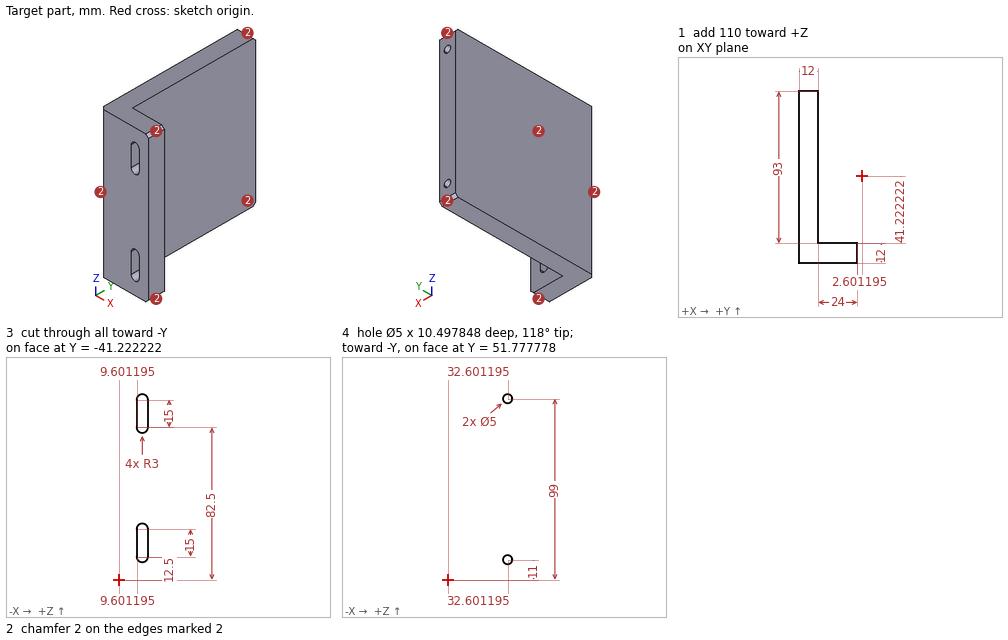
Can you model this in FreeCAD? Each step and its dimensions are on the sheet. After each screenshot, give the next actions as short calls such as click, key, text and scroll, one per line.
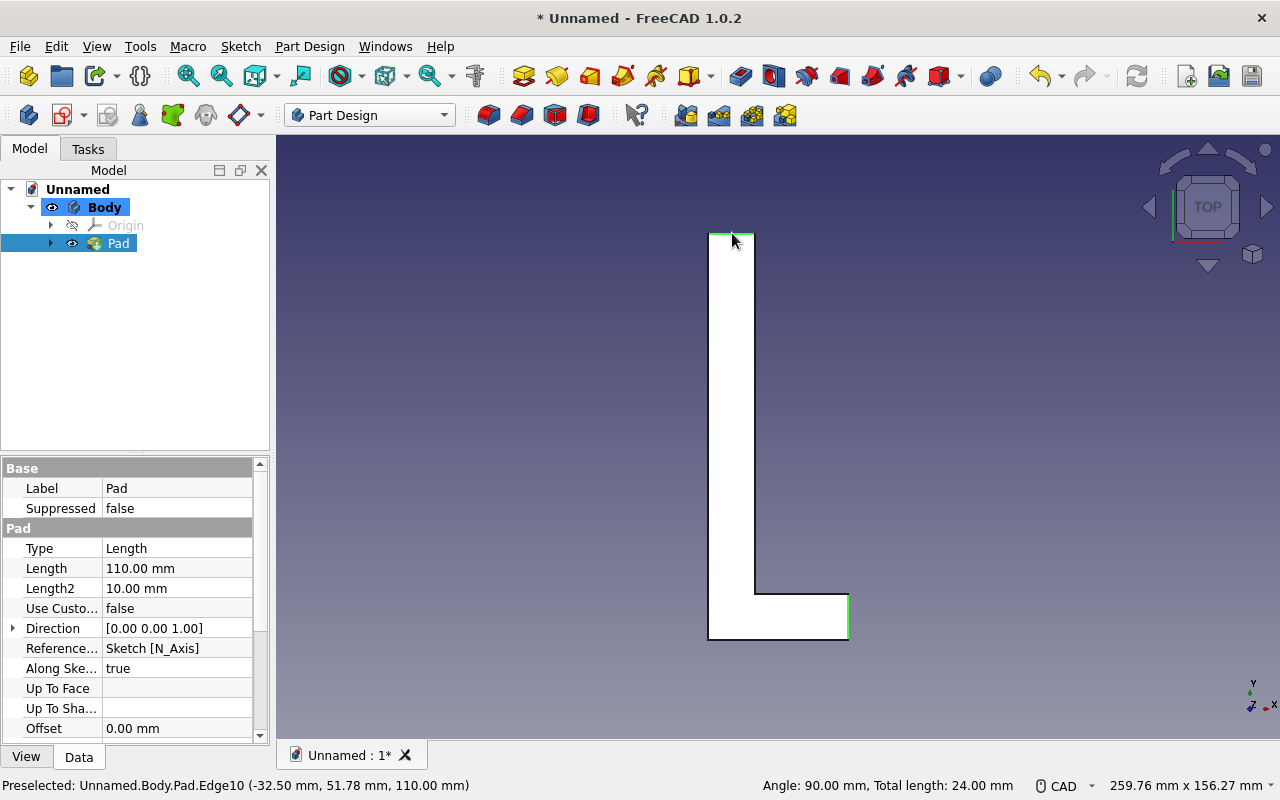
key(1)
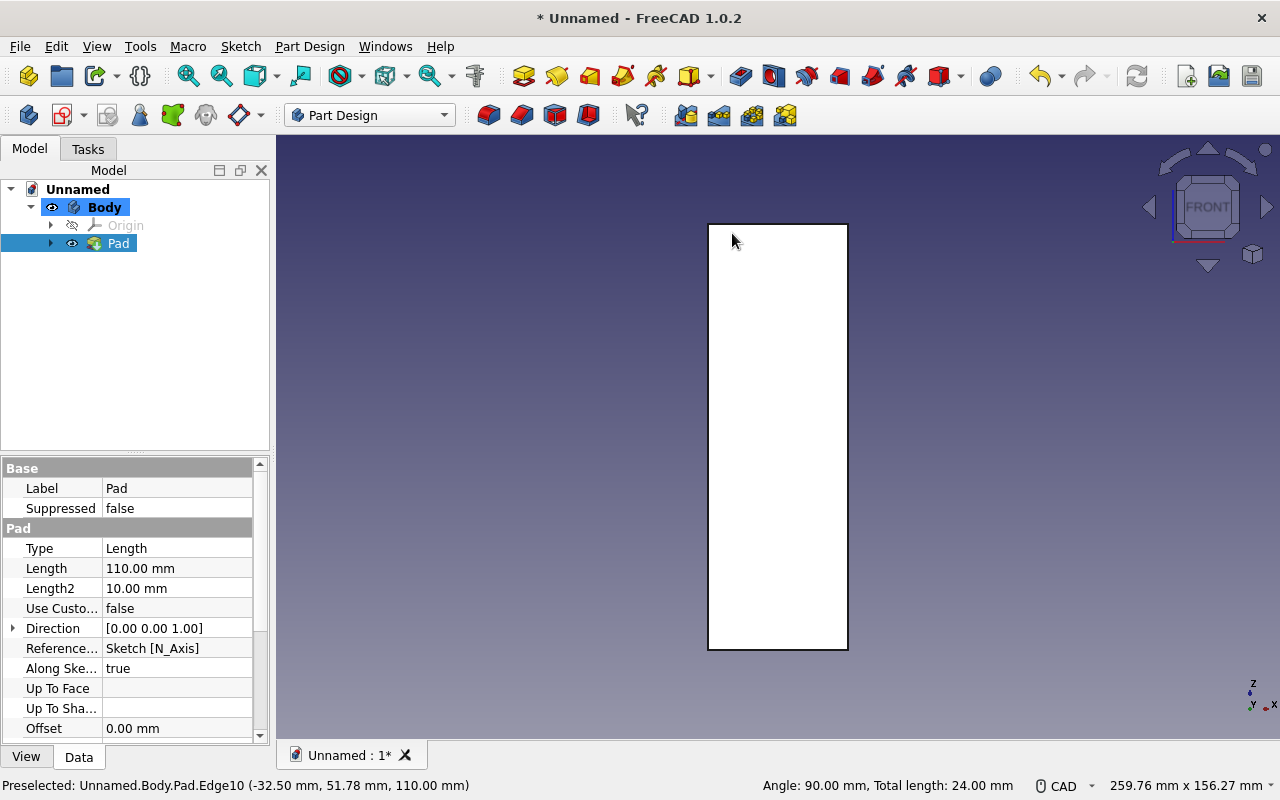
click(708, 436, ctrl)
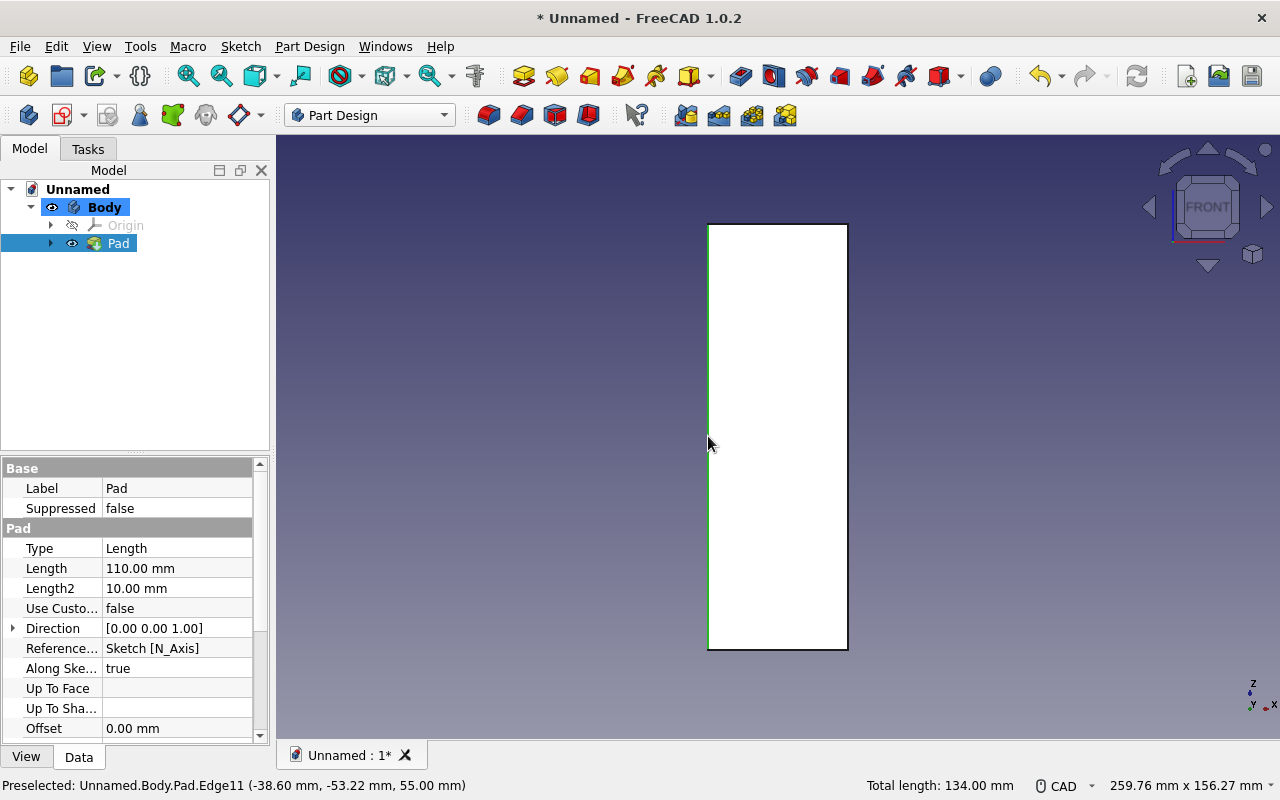
key(3)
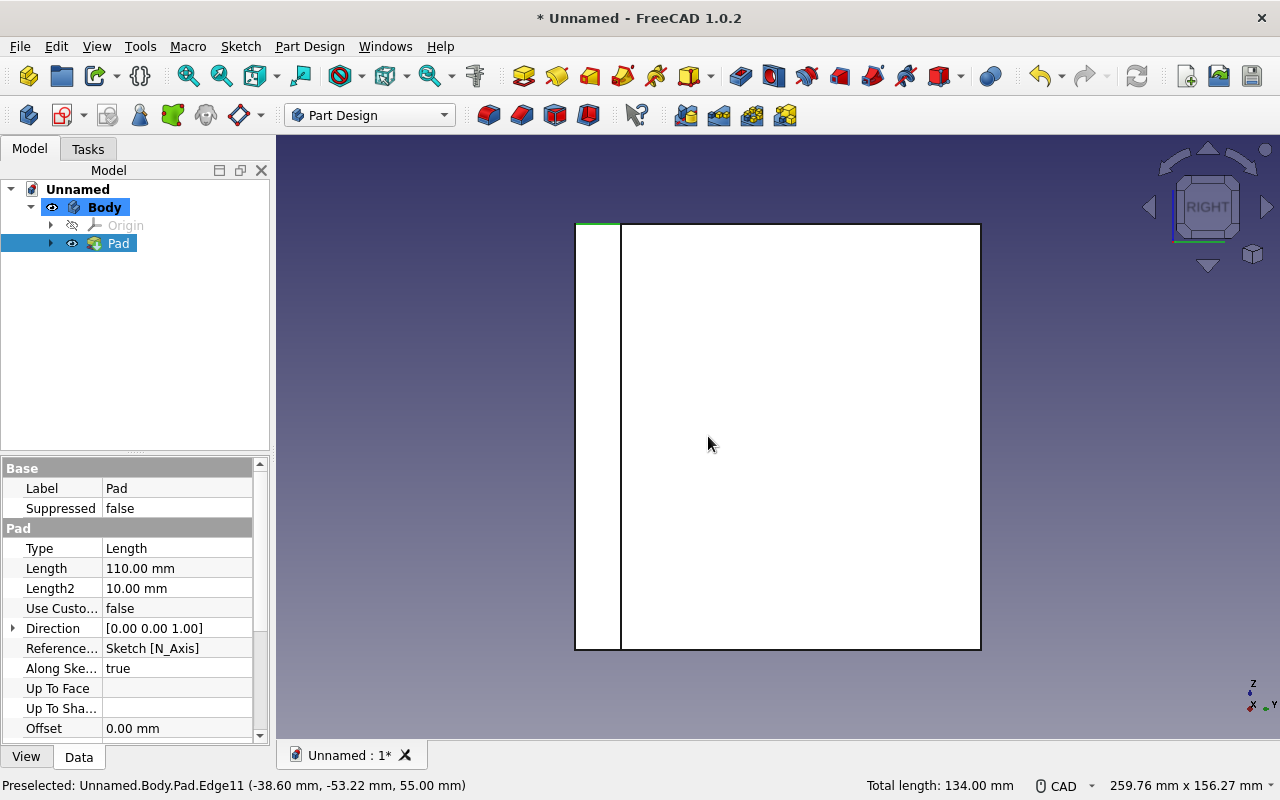
click(598, 649, ctrl)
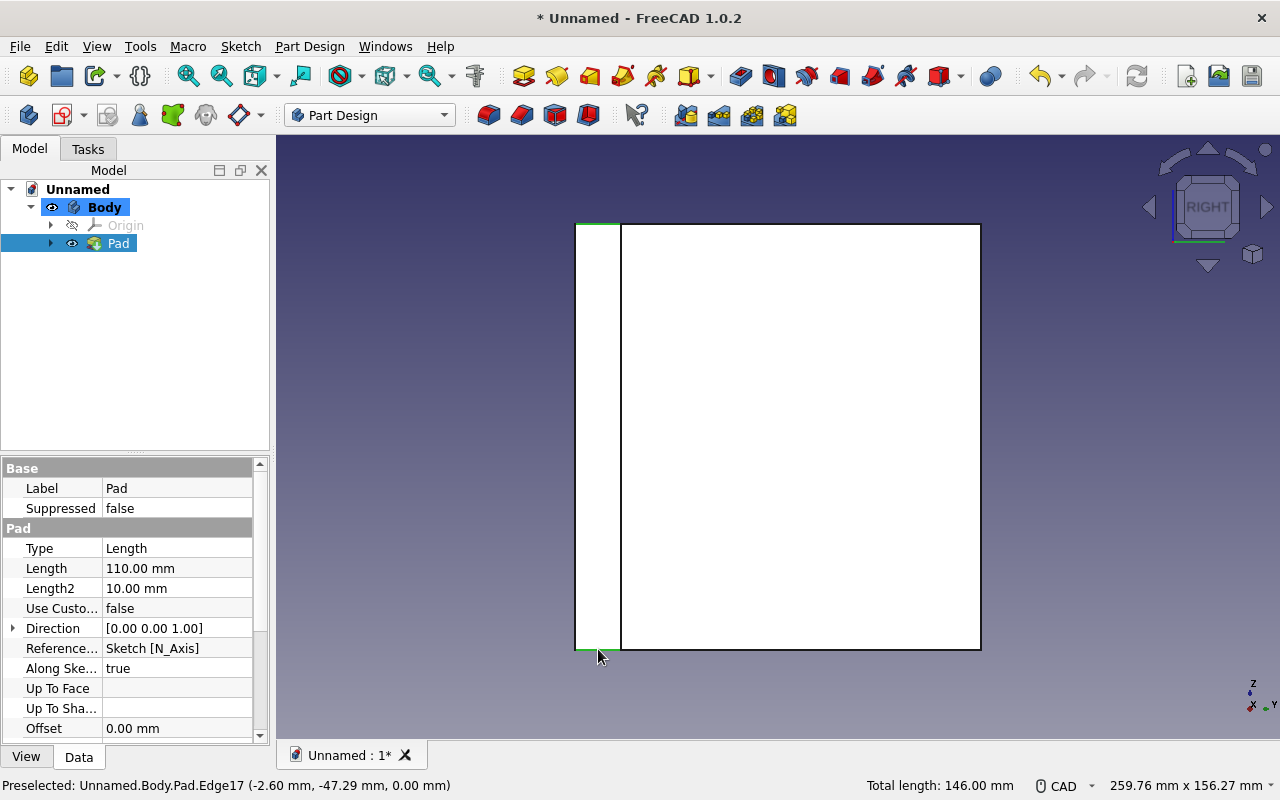
key(5)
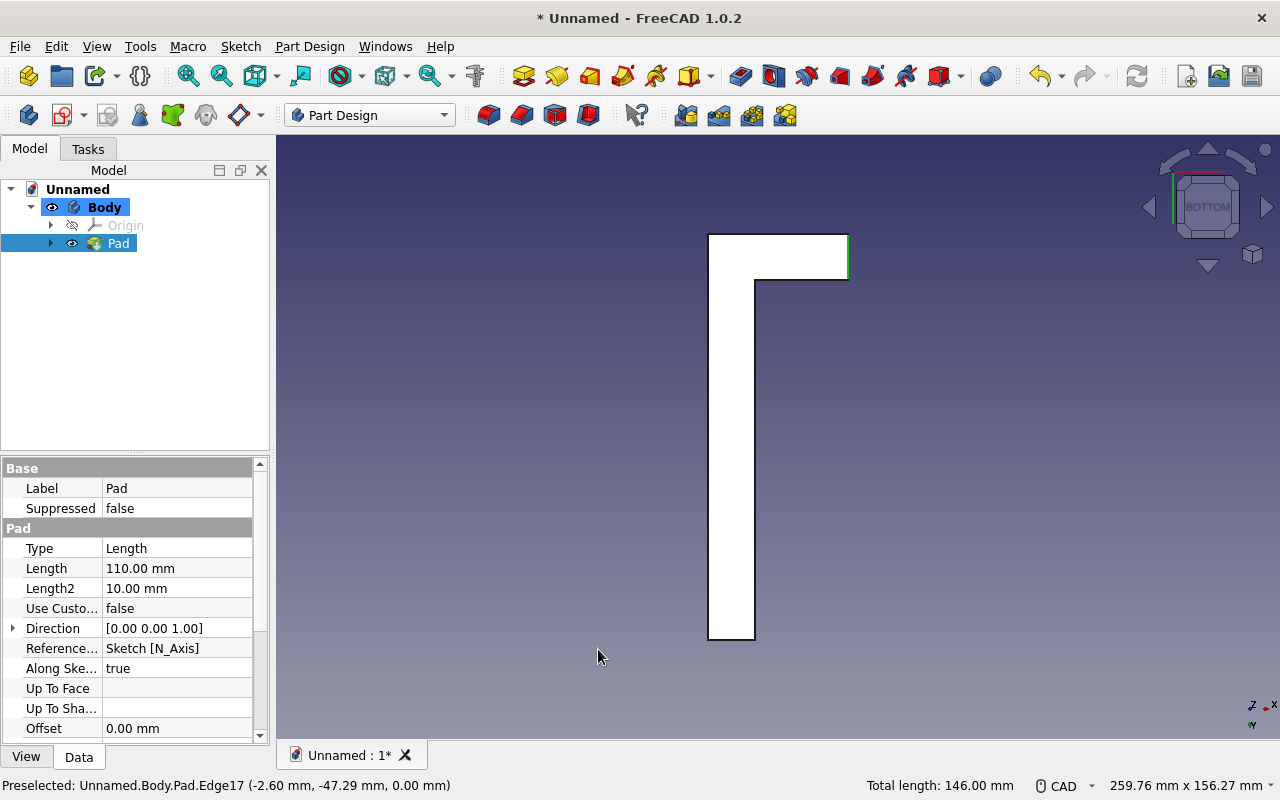
click(732, 639, ctrl)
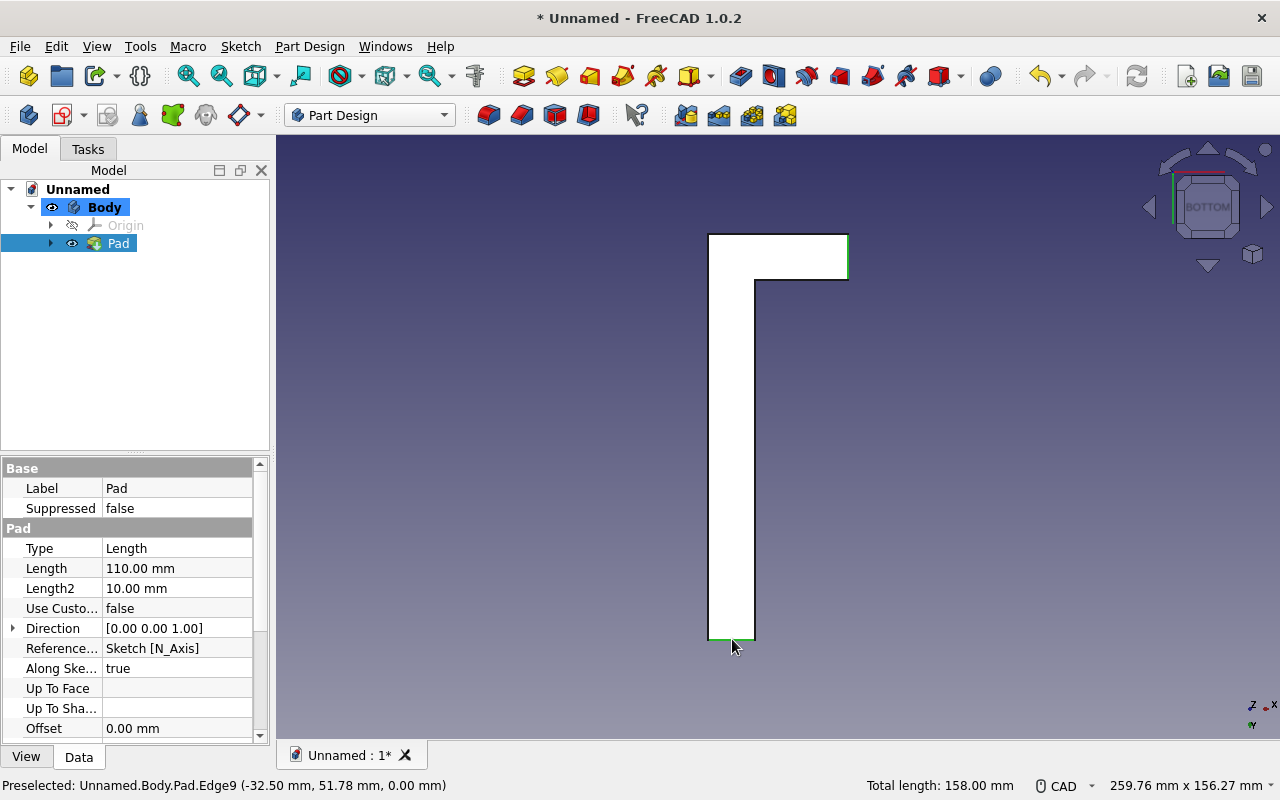
click(522, 116)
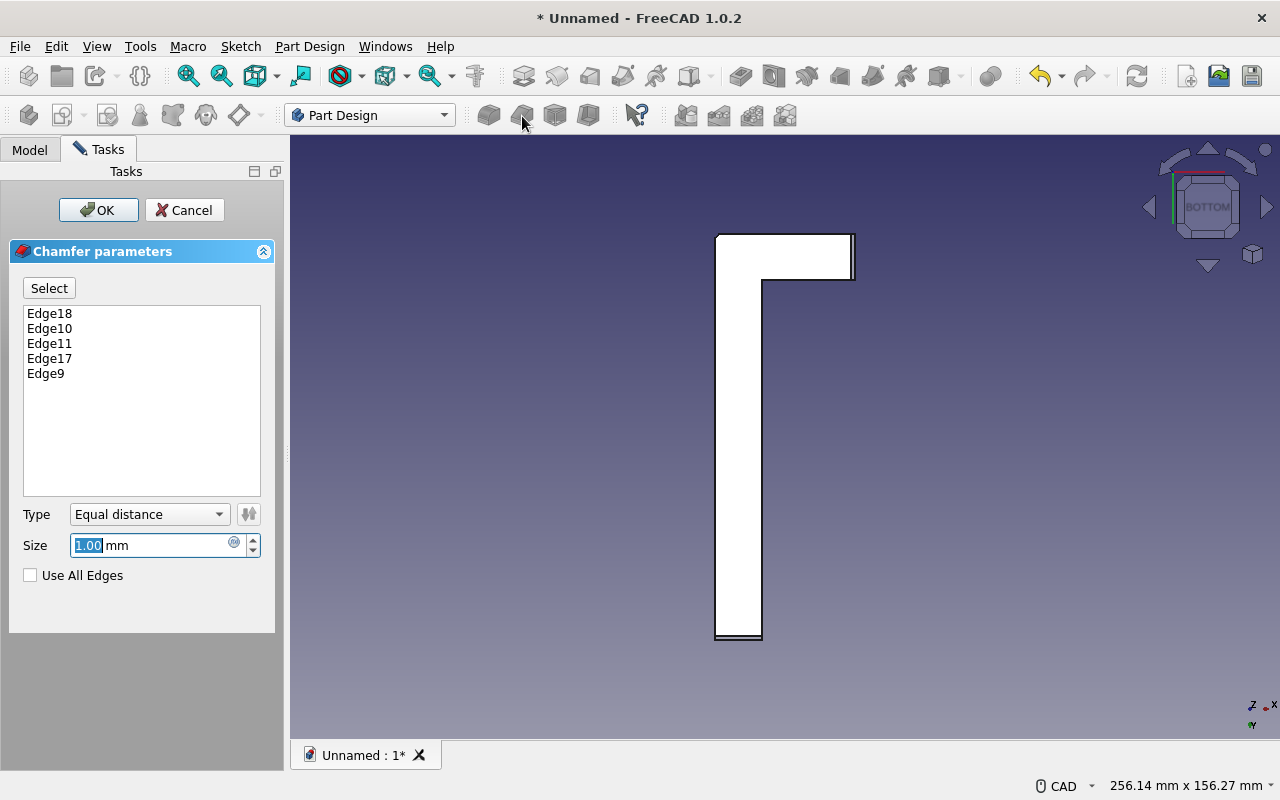
text(2)
key(Tab)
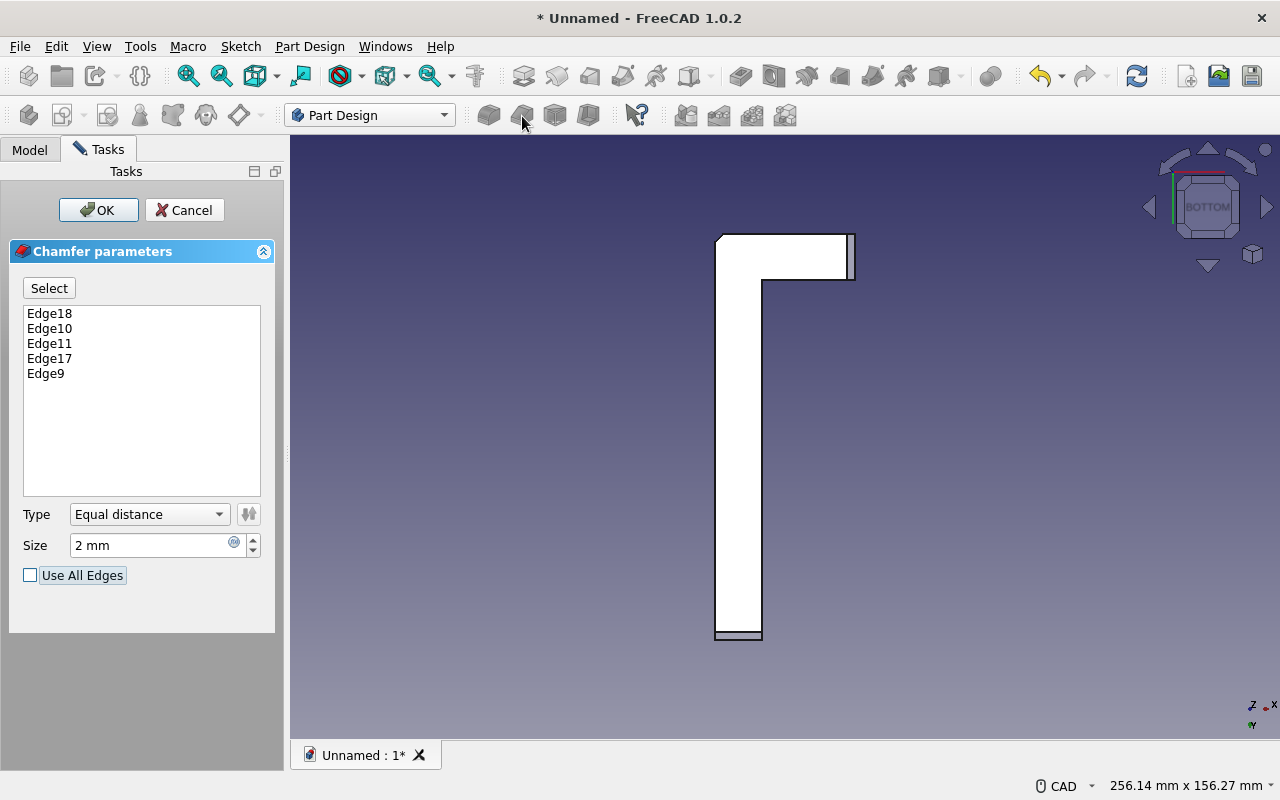
click(99, 210)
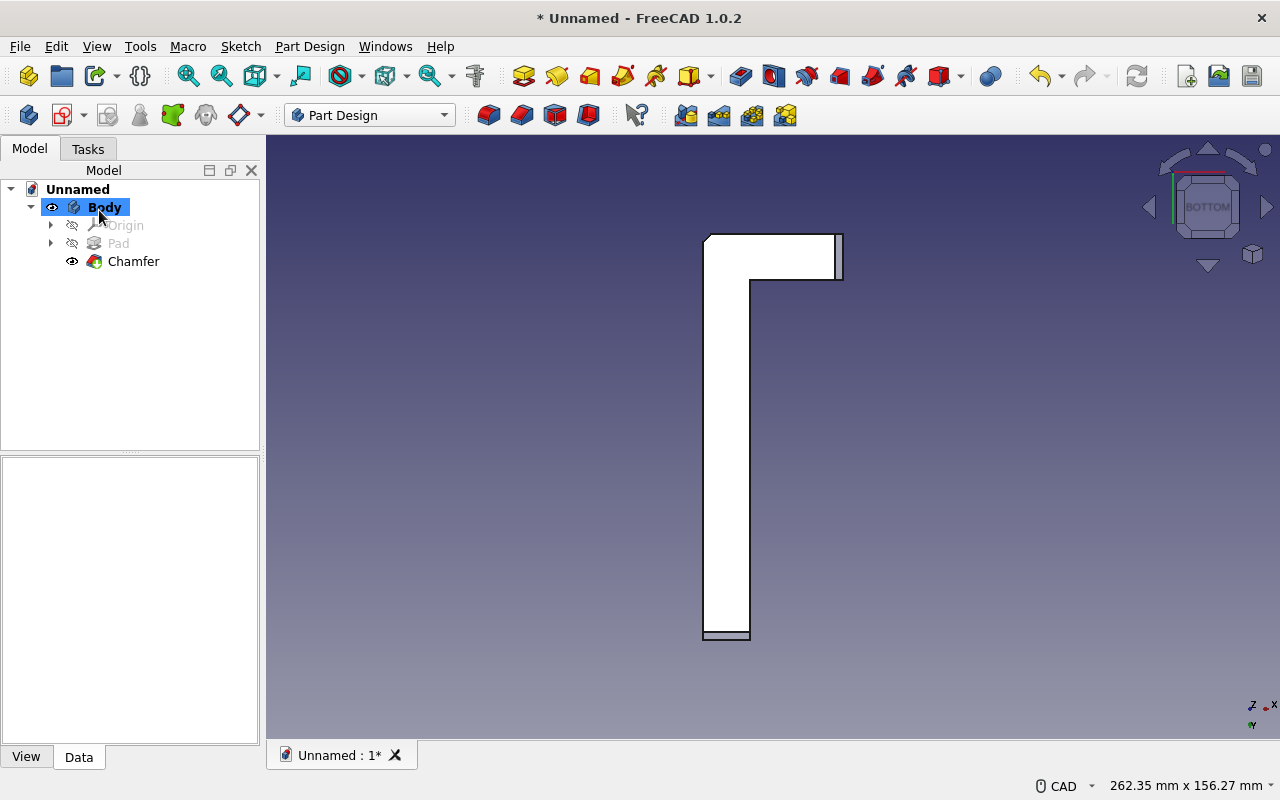
key(4)